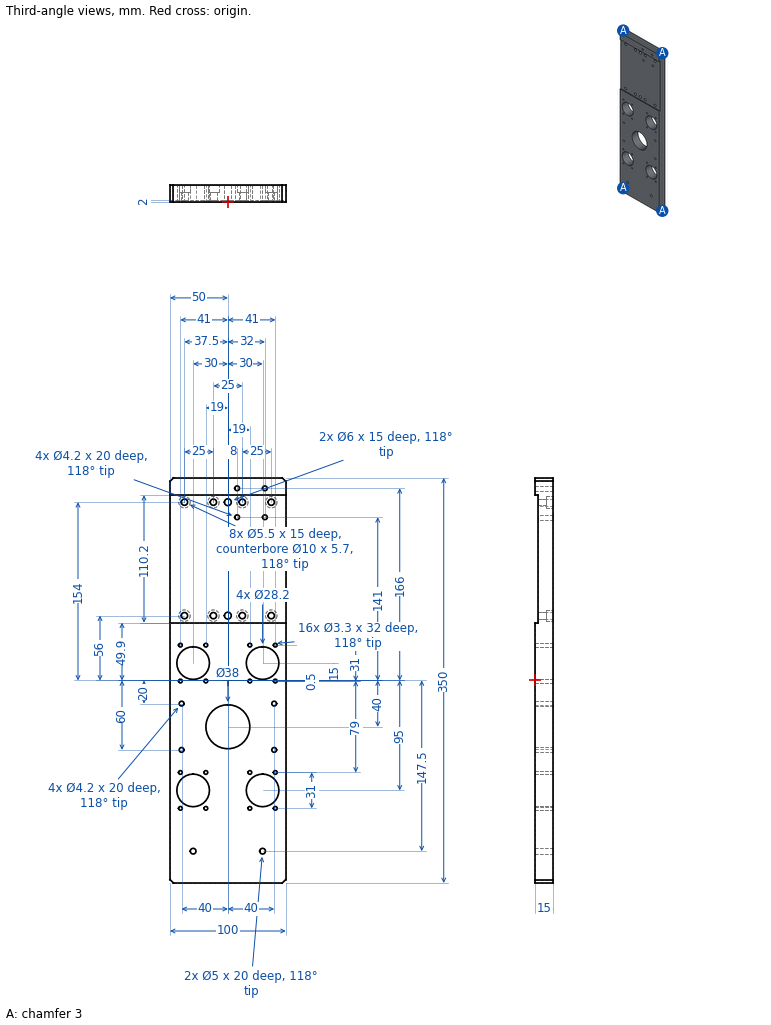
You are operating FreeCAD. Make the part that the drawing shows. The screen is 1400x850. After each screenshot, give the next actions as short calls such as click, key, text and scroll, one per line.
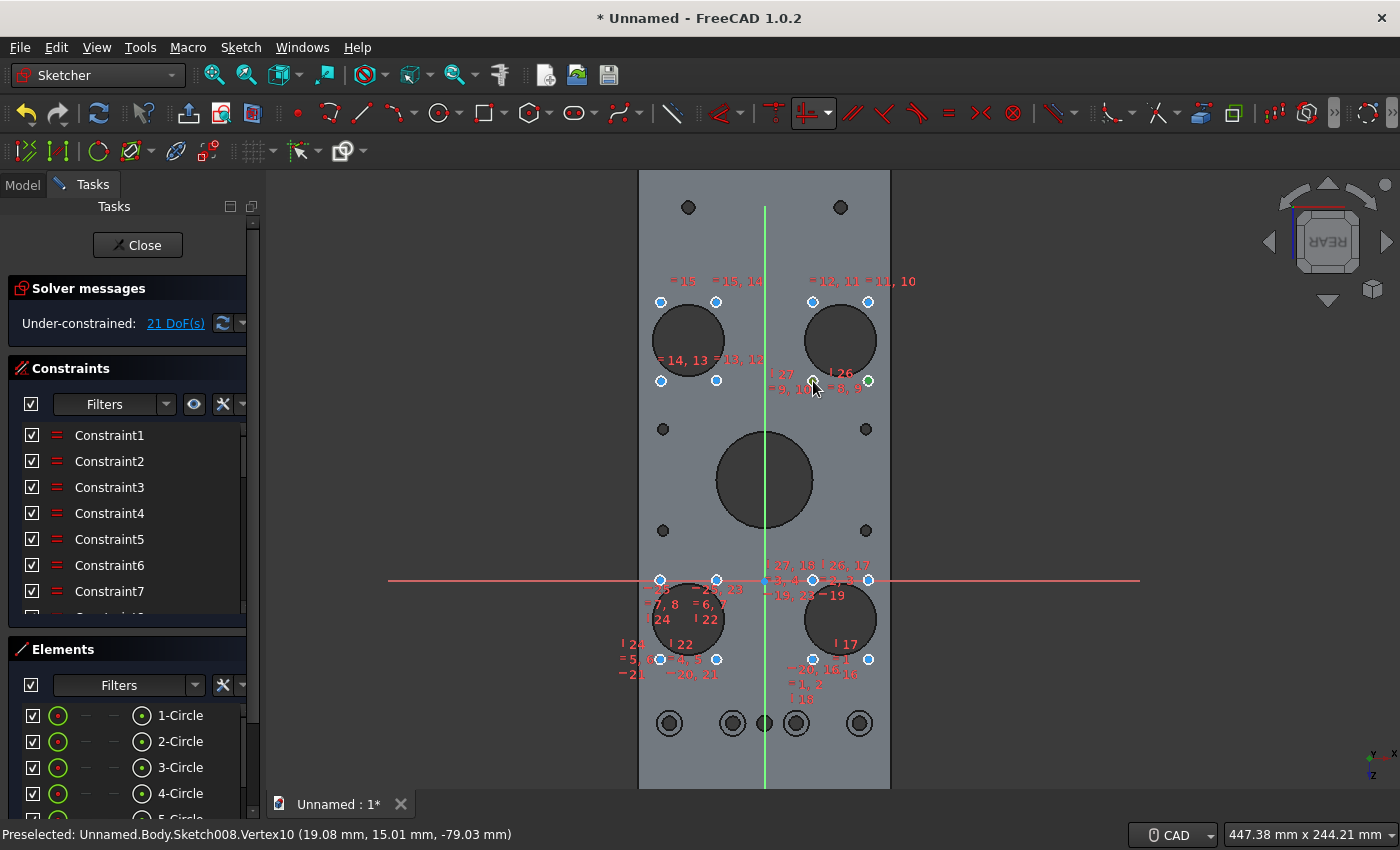
key(h)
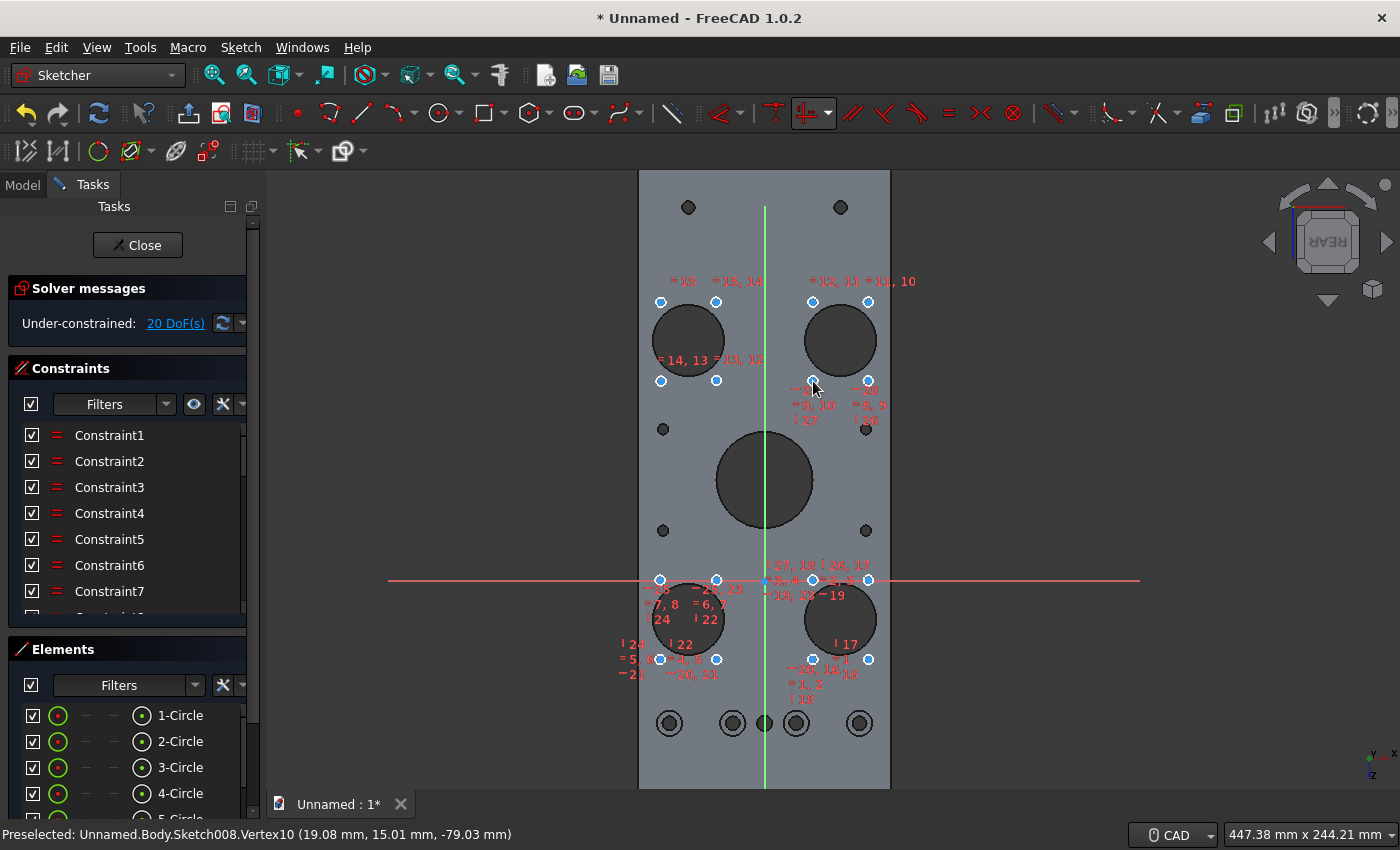
click(868, 381)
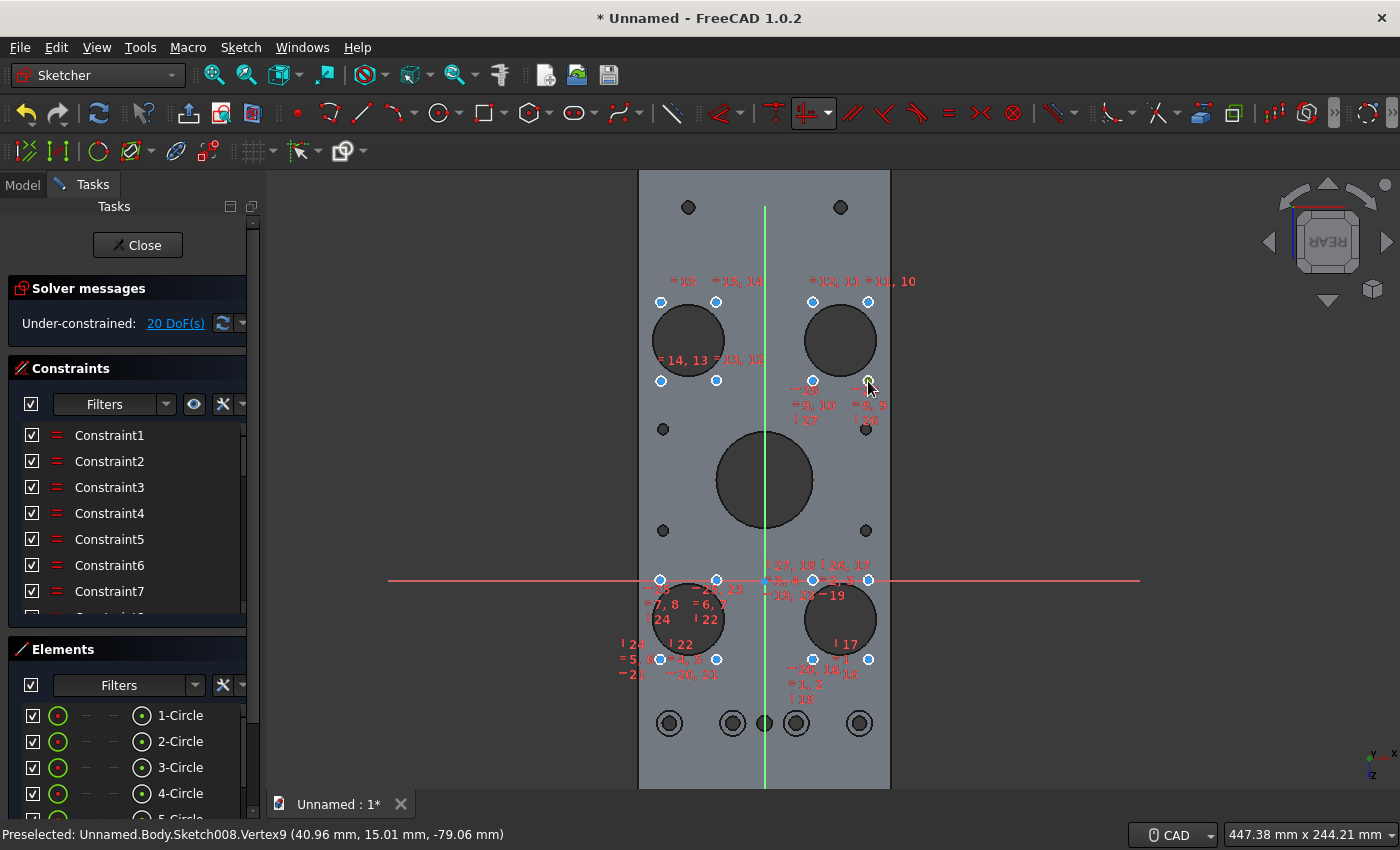
click(868, 302)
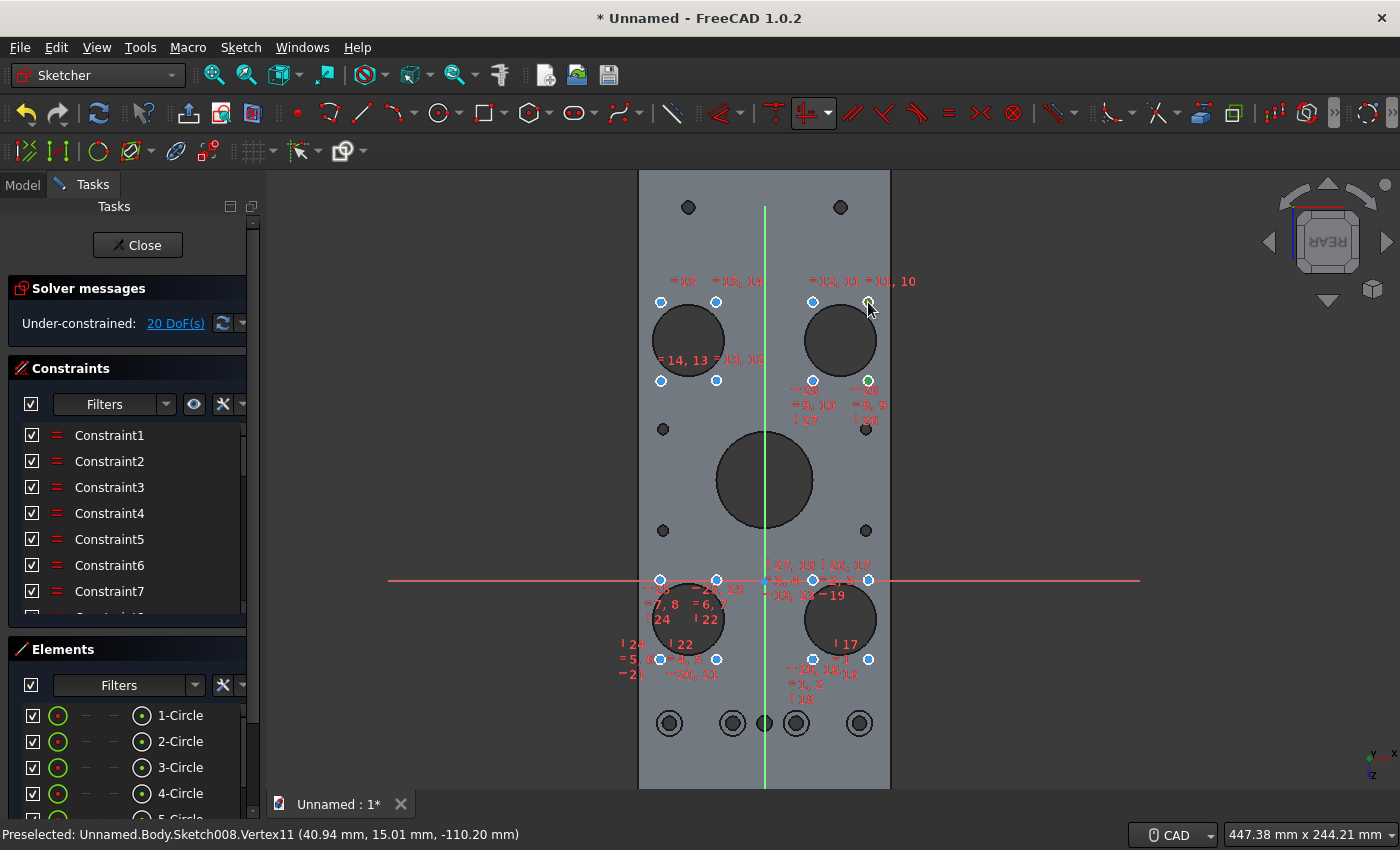
key(v)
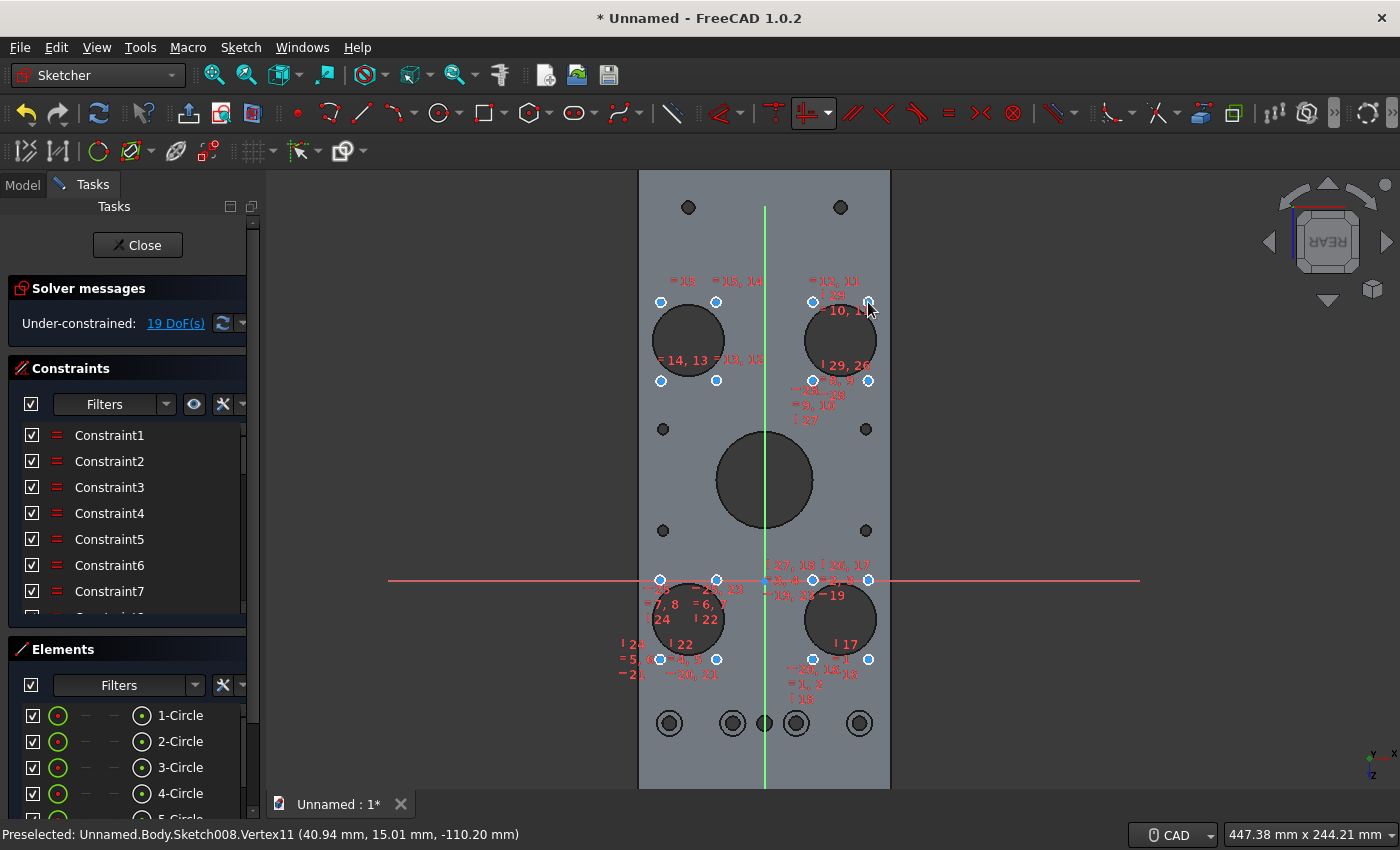
click(813, 381)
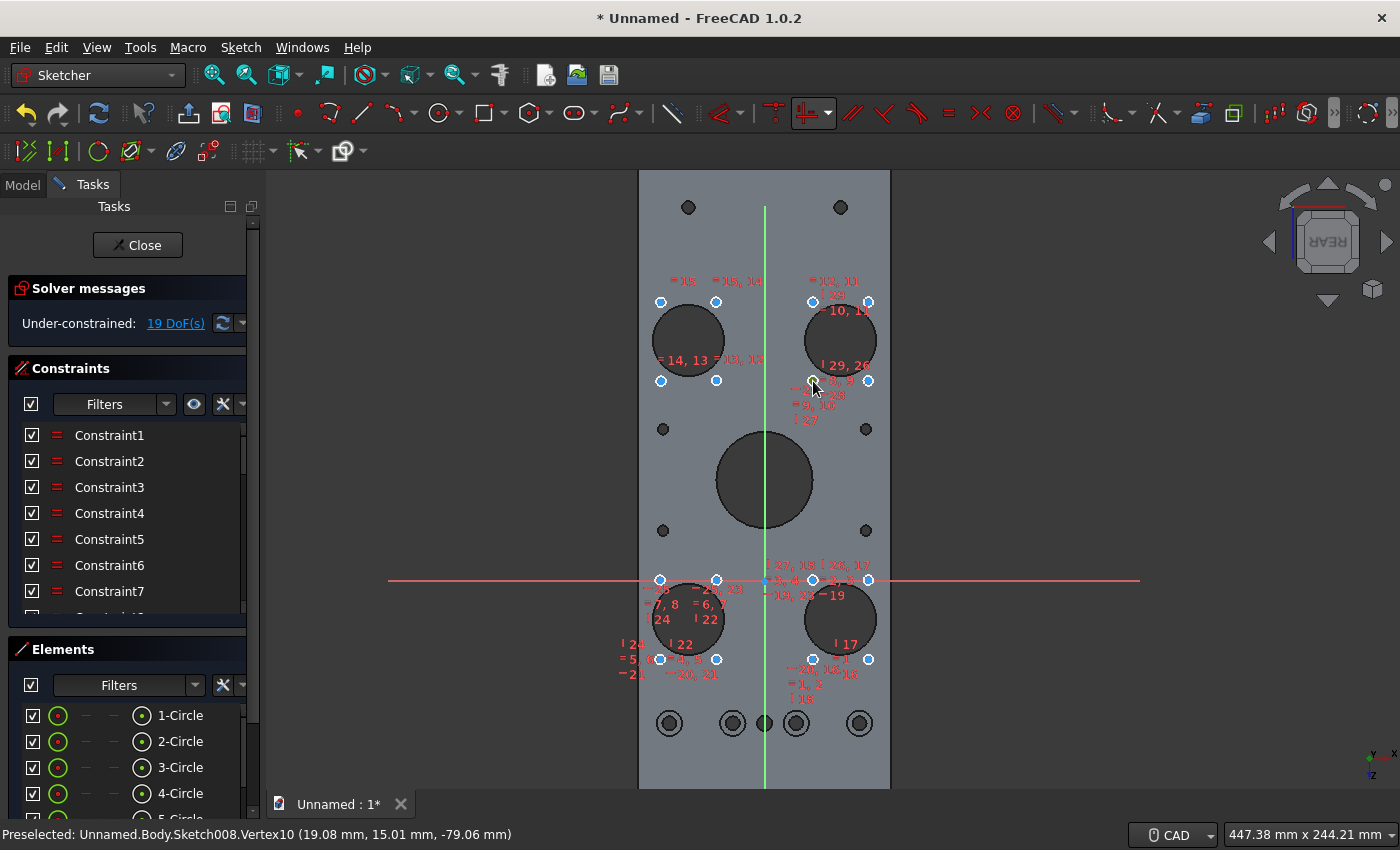
click(813, 302)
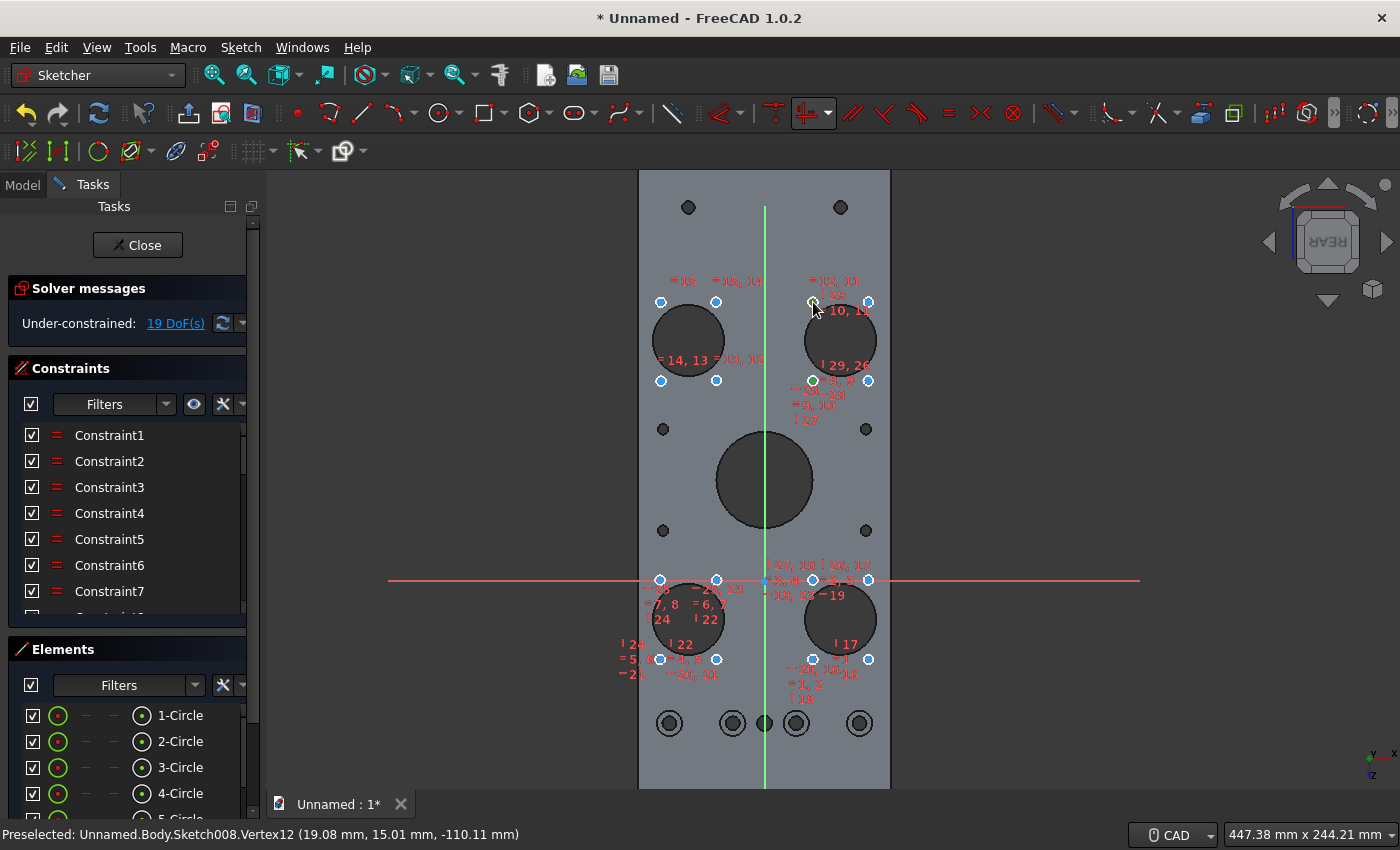
key(v)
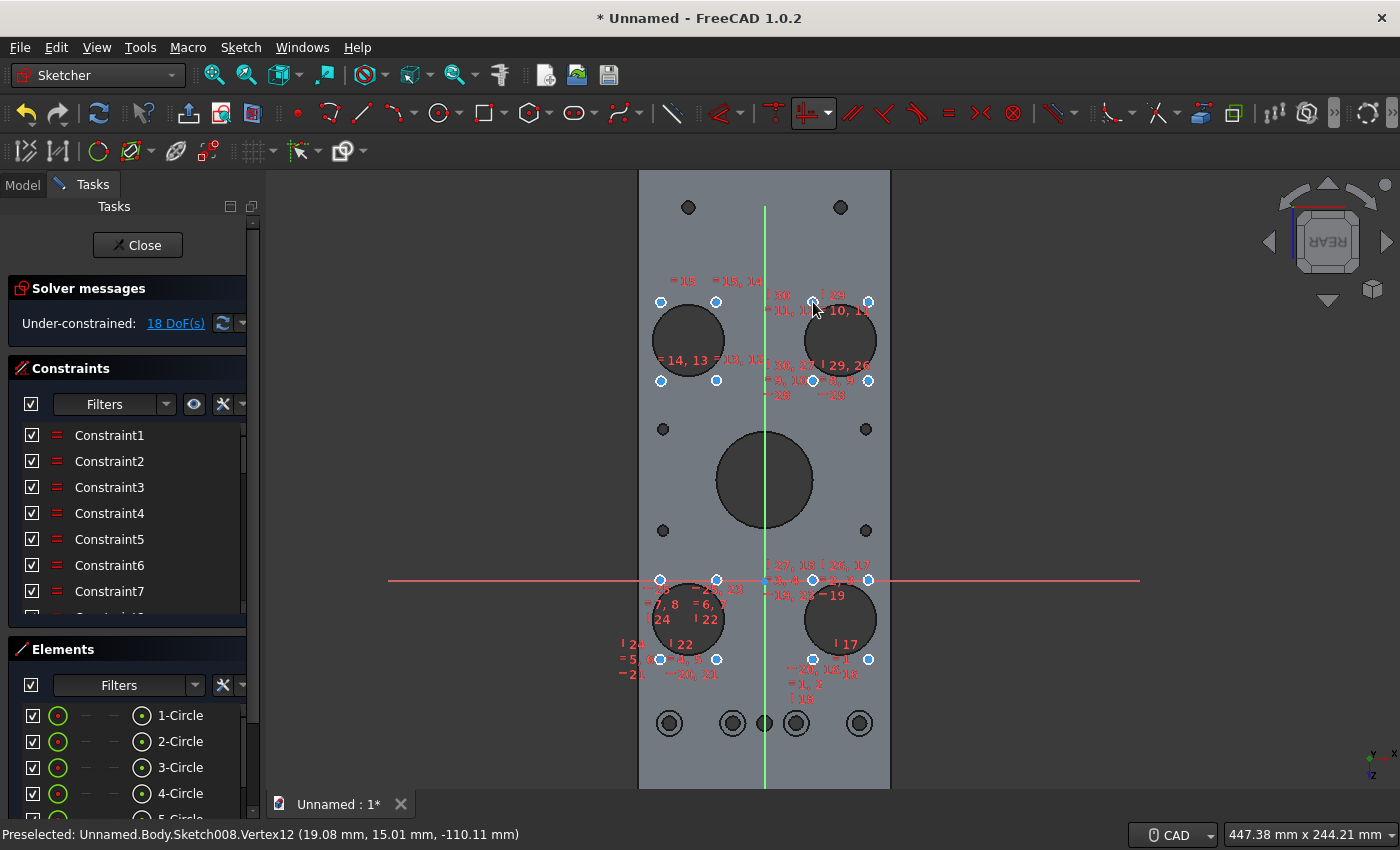
click(870, 304)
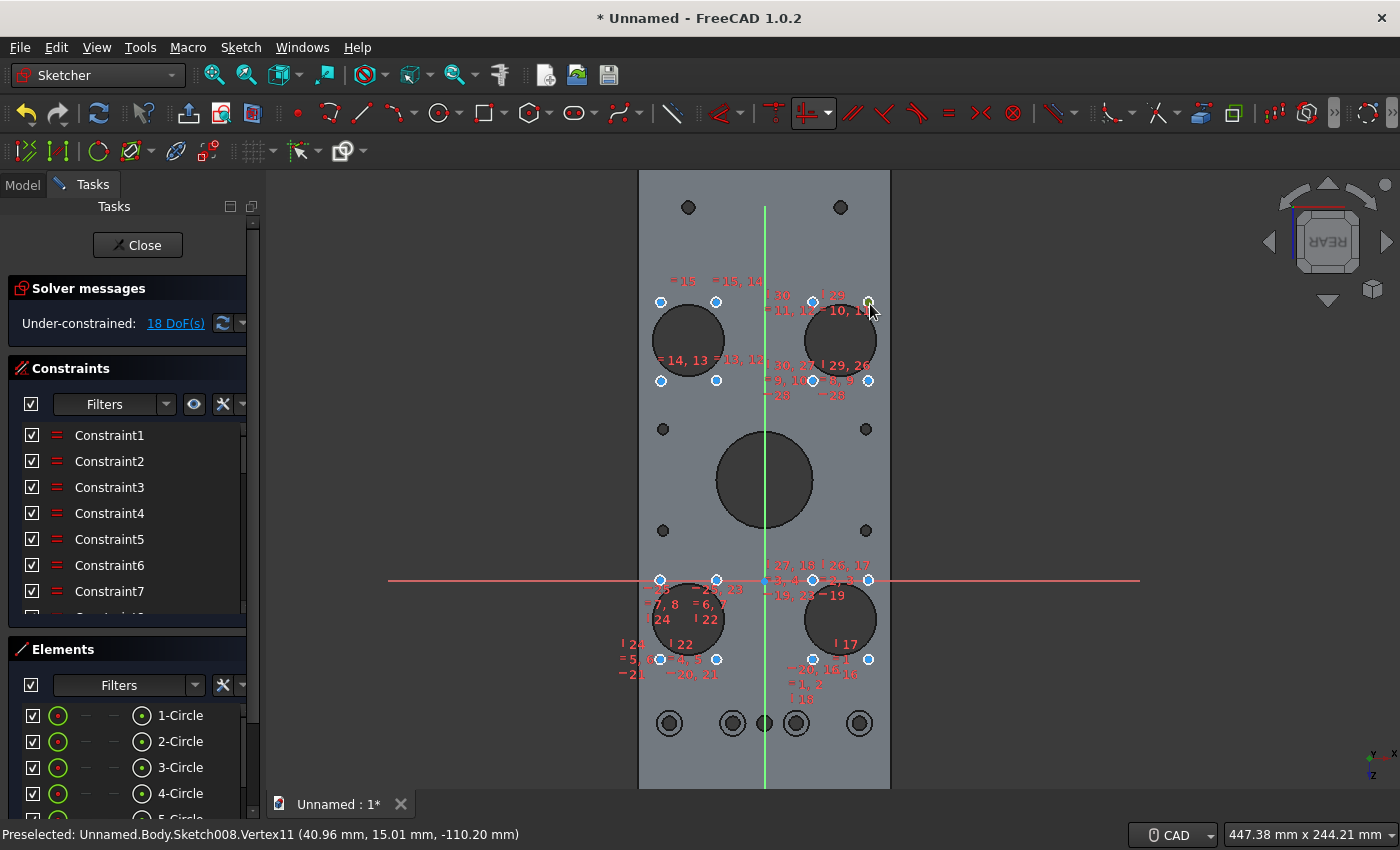
click(815, 304)